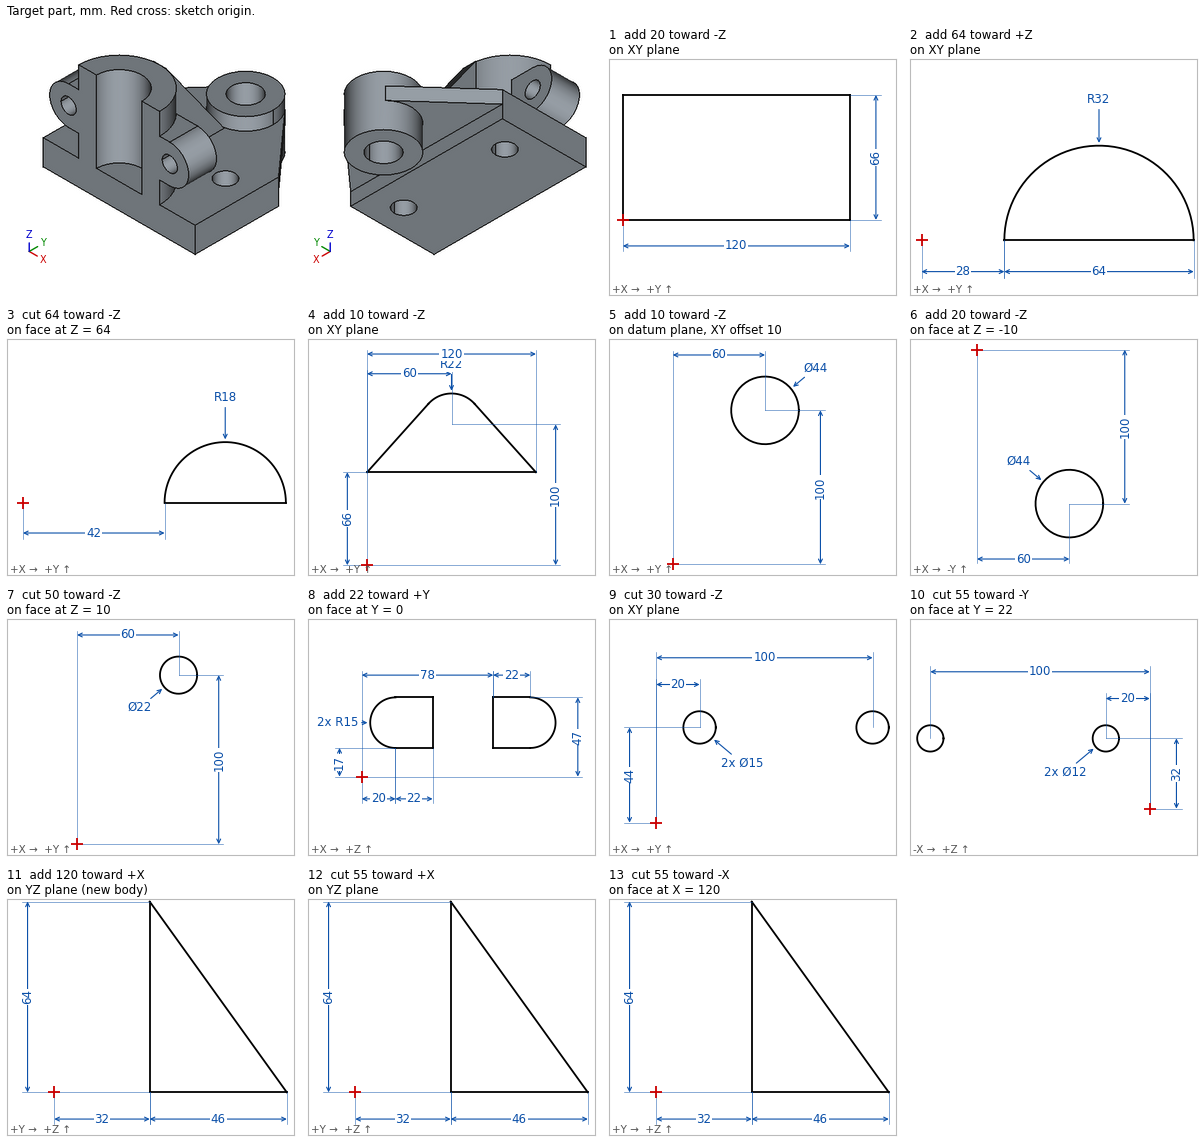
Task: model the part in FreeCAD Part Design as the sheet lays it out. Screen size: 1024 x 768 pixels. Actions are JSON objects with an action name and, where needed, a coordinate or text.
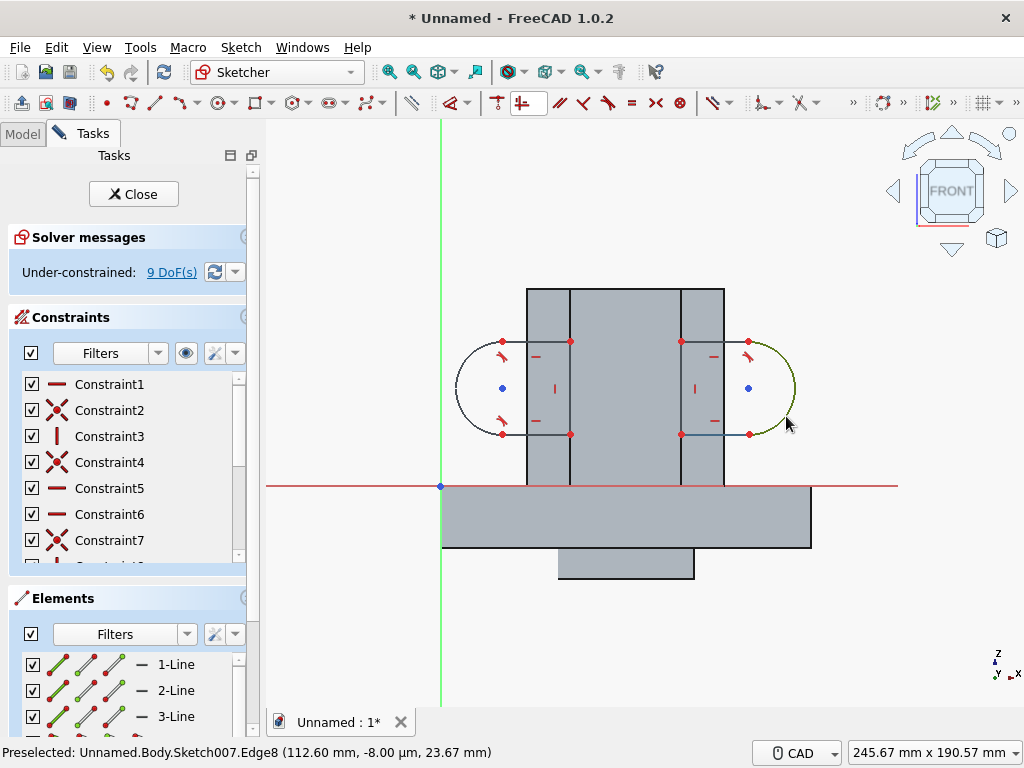
{"action": "left_click", "coordinate": [608, 104]}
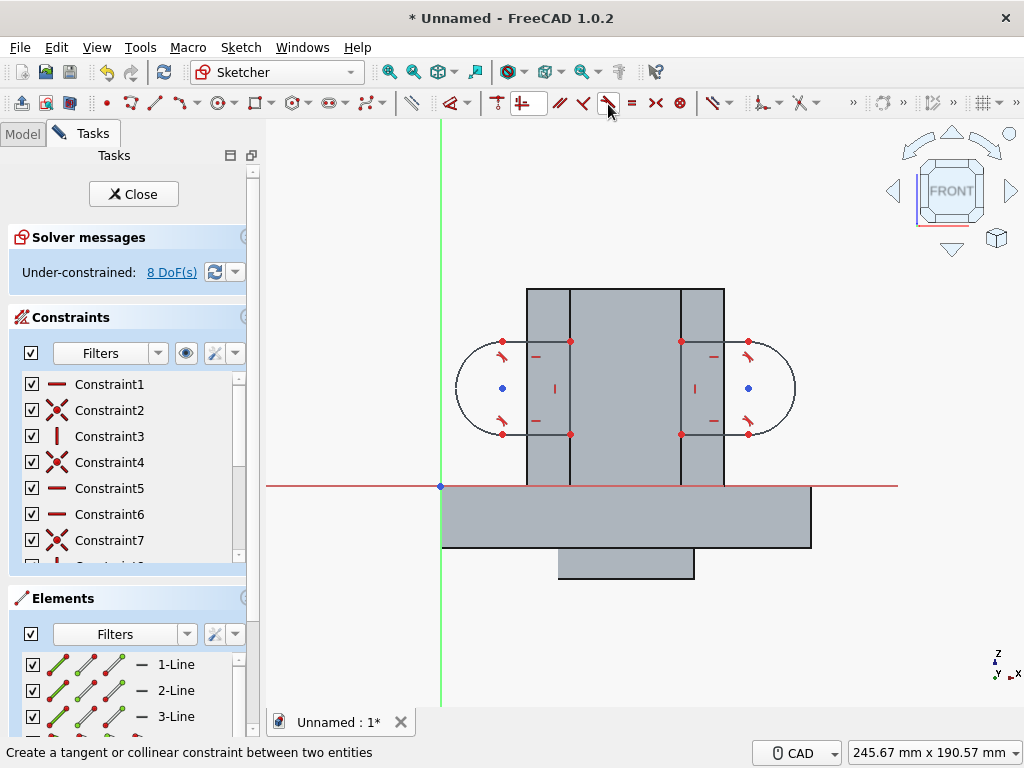
{"action": "left_click", "coordinate": [465, 361]}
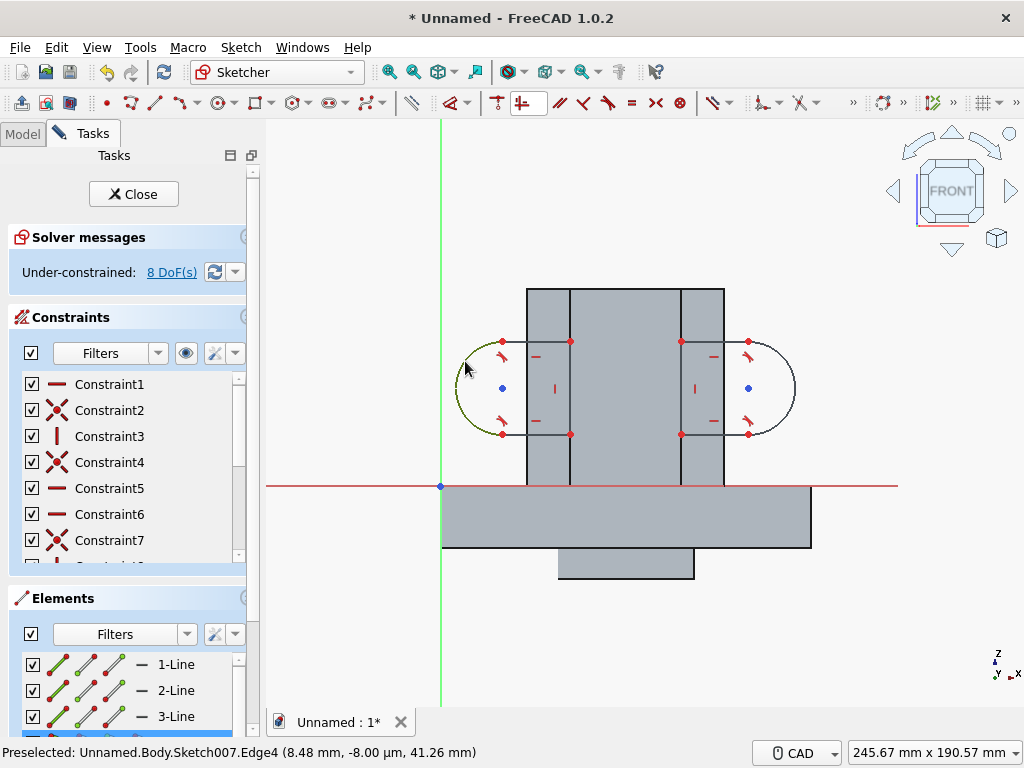
{"action": "left_click", "coordinate": [786, 416]}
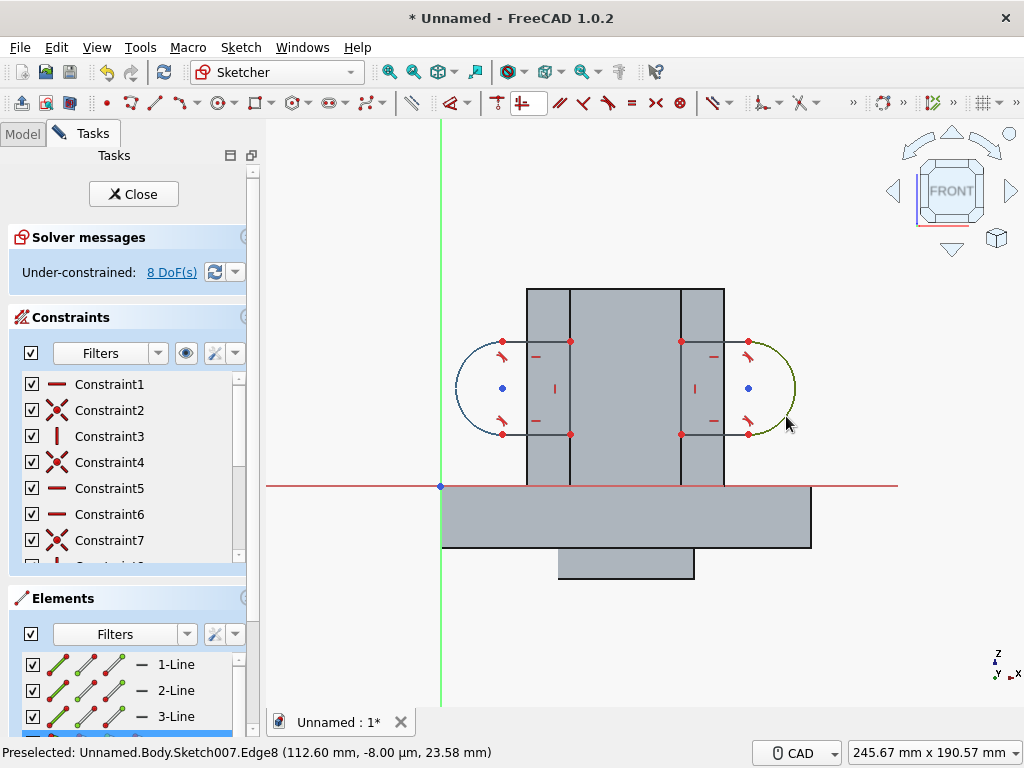
{"action": "left_click", "coordinate": [632, 104]}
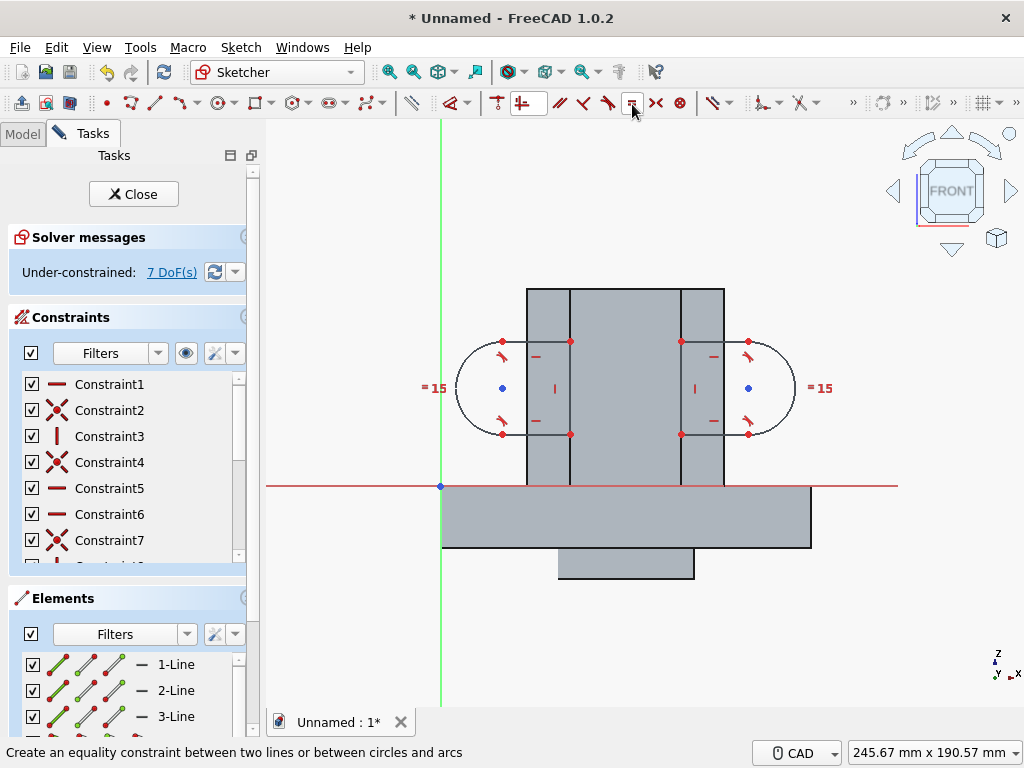
{"action": "left_click", "coordinate": [450, 104]}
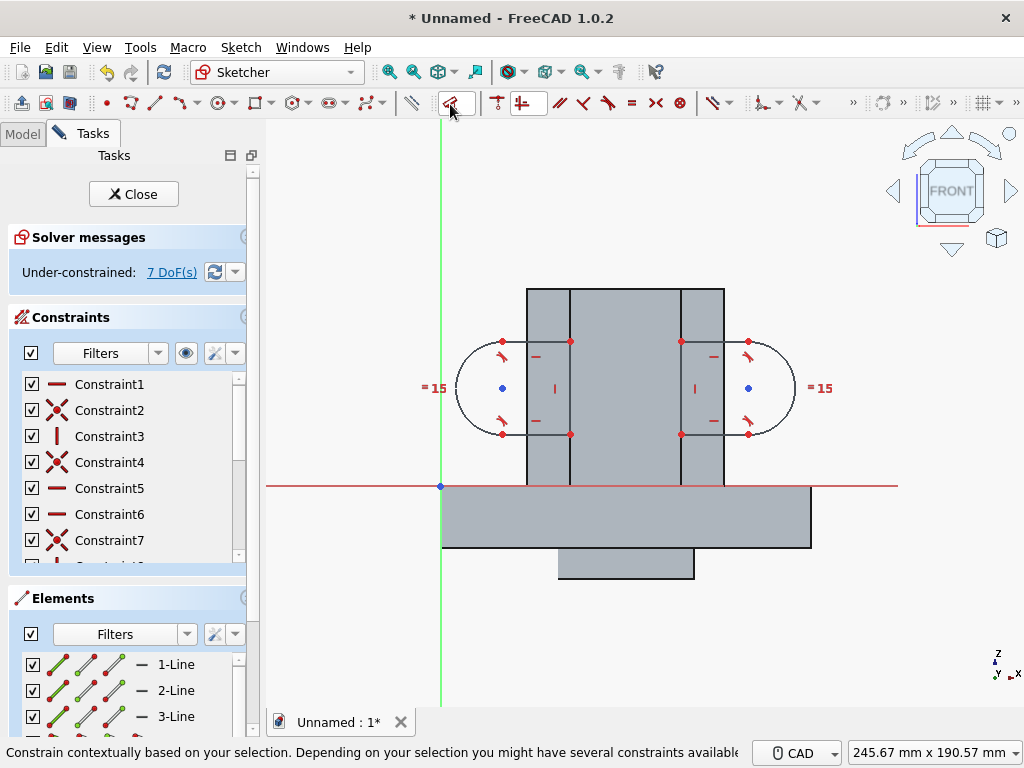
{"action": "left_click", "coordinate": [465, 361]}
{"action": "left_click", "coordinate": [469, 317]}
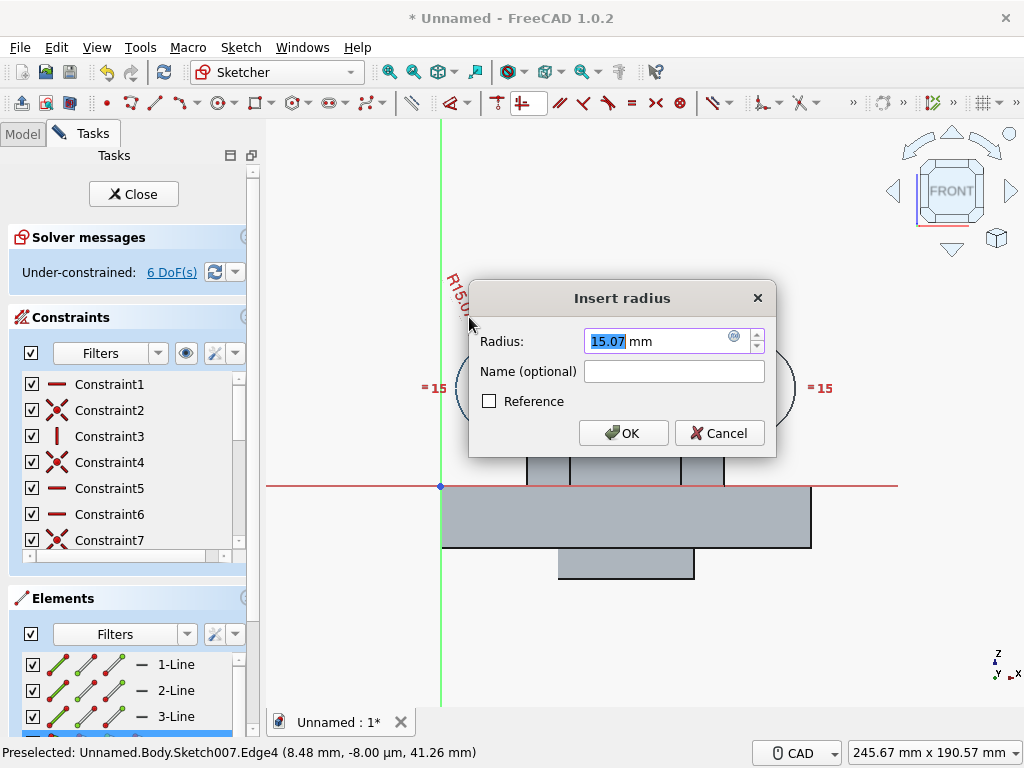
{"action": "type", "text": "15"}
{"action": "key", "text": "Return"}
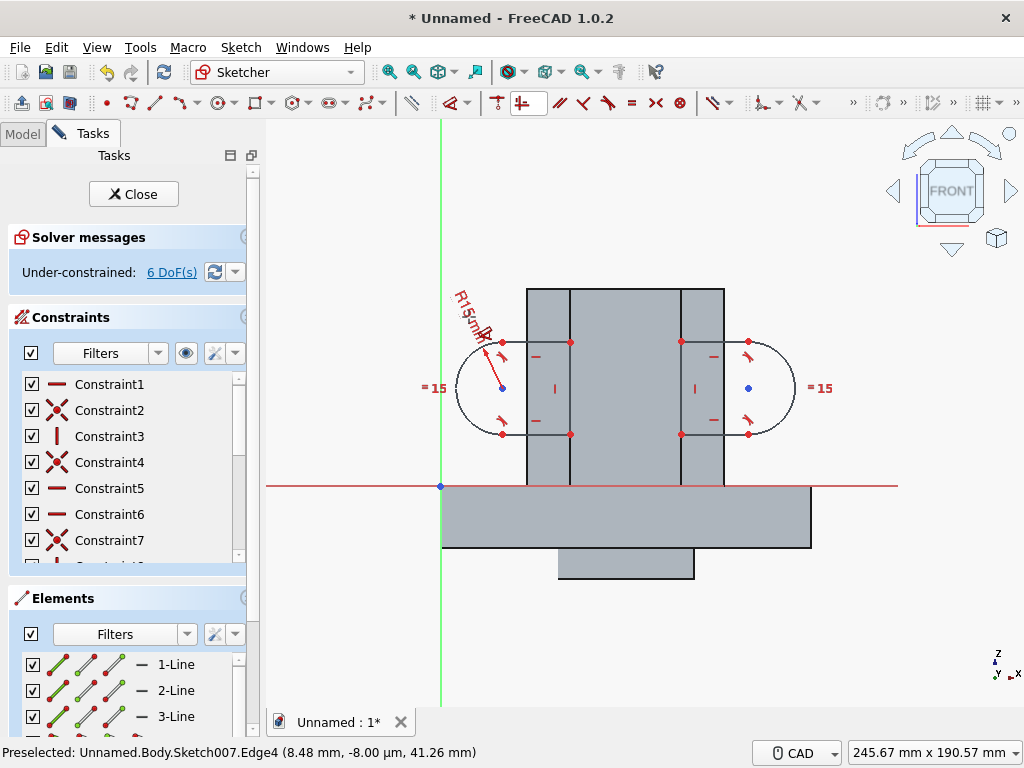
{"action": "left_click", "coordinate": [523, 435]}
{"action": "left_click", "coordinate": [536, 469]}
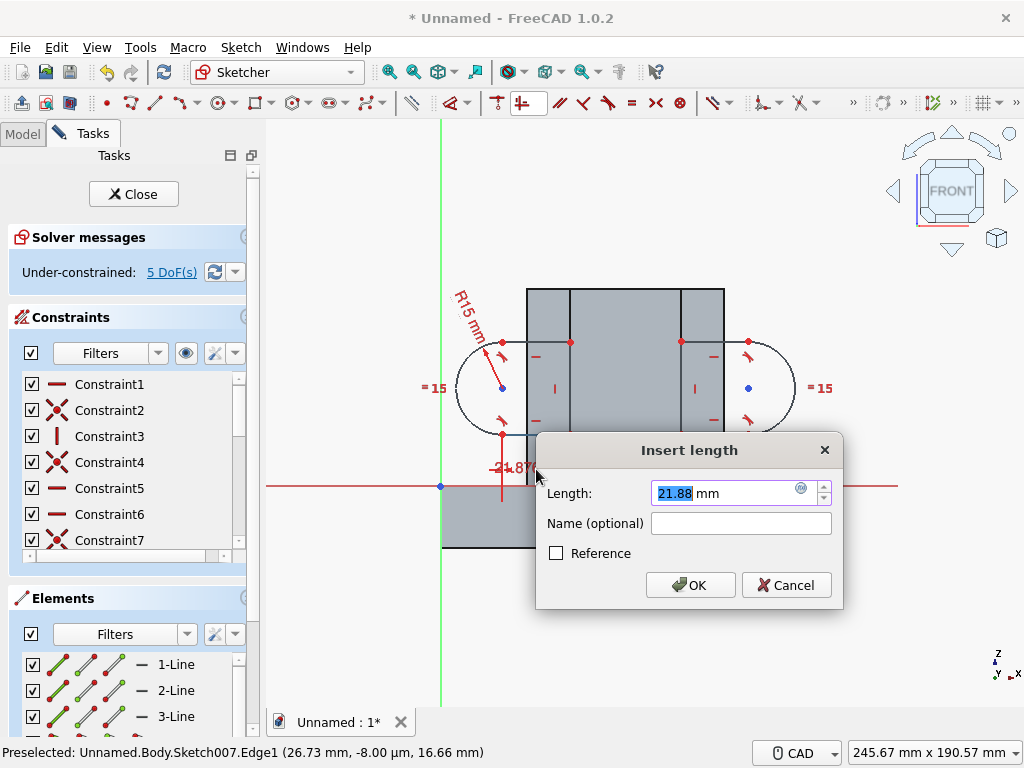
{"action": "type", "text": "22"}
{"action": "key", "text": "Return"}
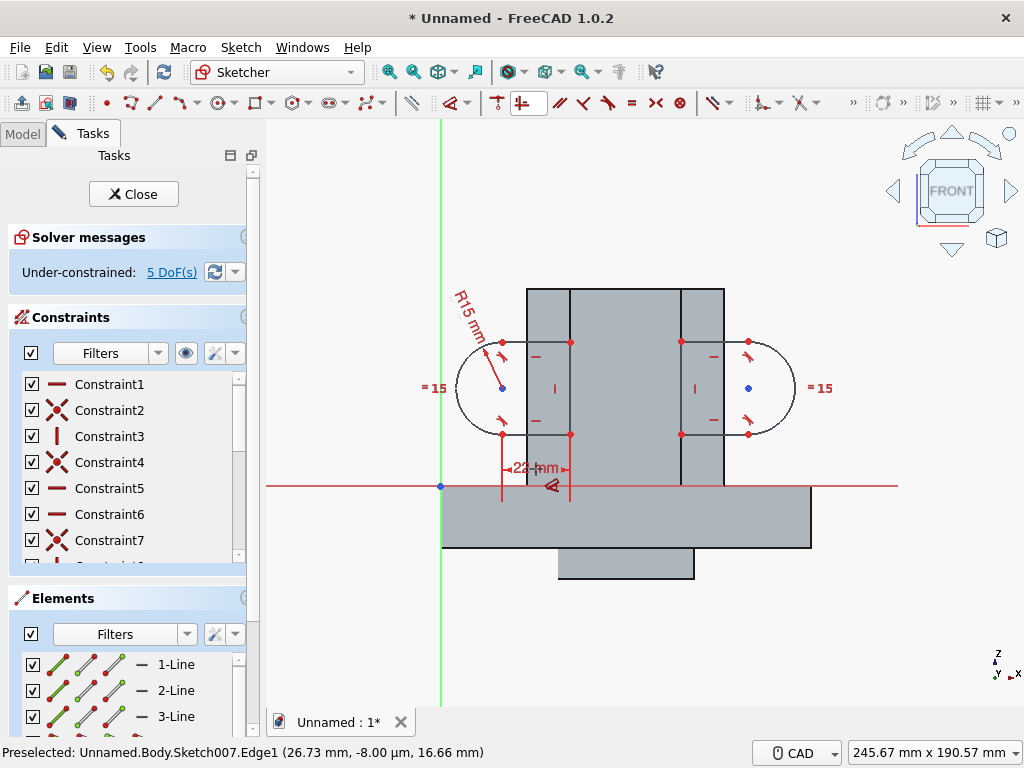
{"action": "left_click", "coordinate": [728, 342]}
{"action": "left_click", "coordinate": [715, 308]}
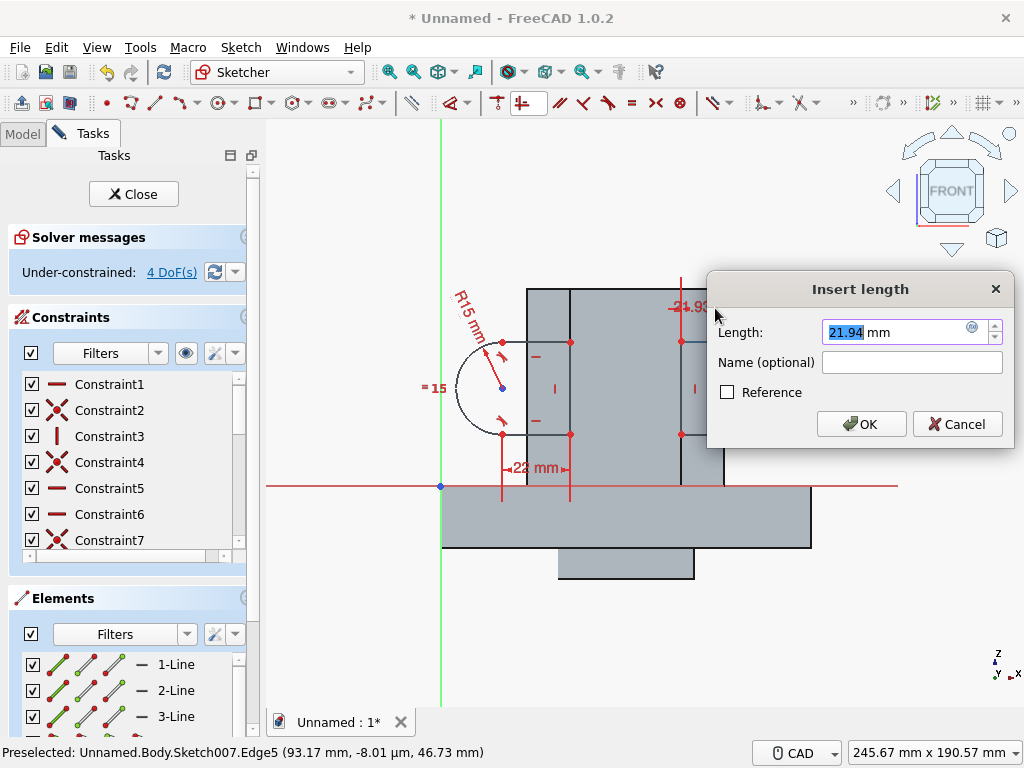
{"action": "type", "text": "22"}
{"action": "key", "text": "Return"}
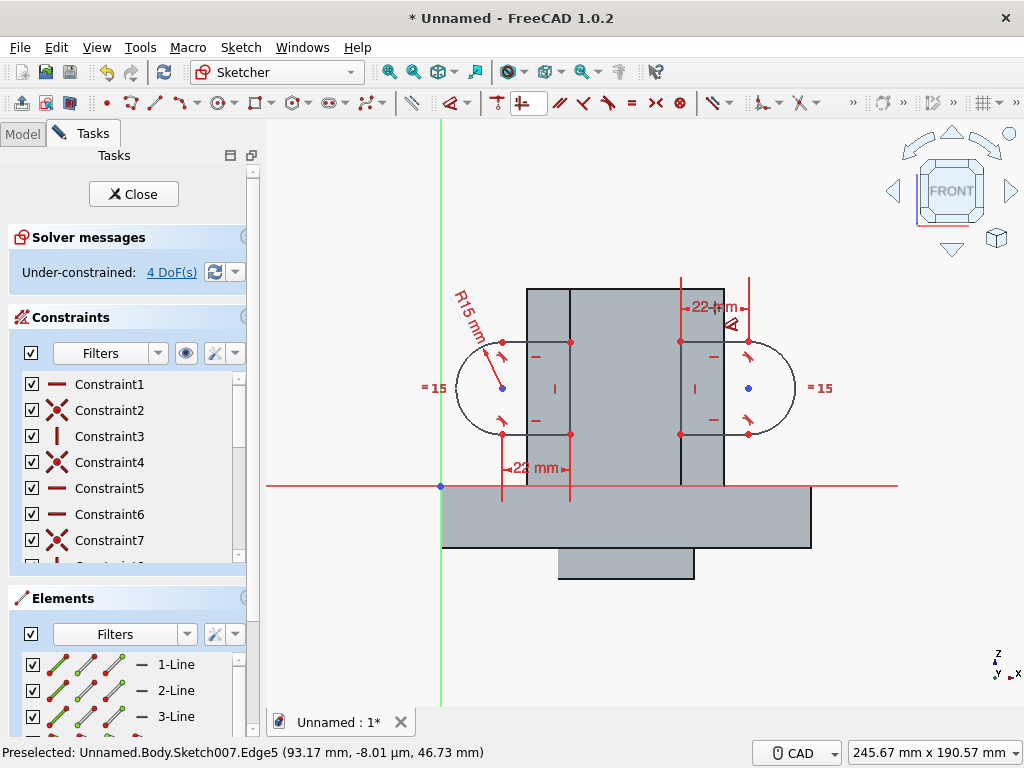
{"action": "left_click", "coordinate": [502, 435]}
{"action": "left_click", "coordinate": [472, 520]}